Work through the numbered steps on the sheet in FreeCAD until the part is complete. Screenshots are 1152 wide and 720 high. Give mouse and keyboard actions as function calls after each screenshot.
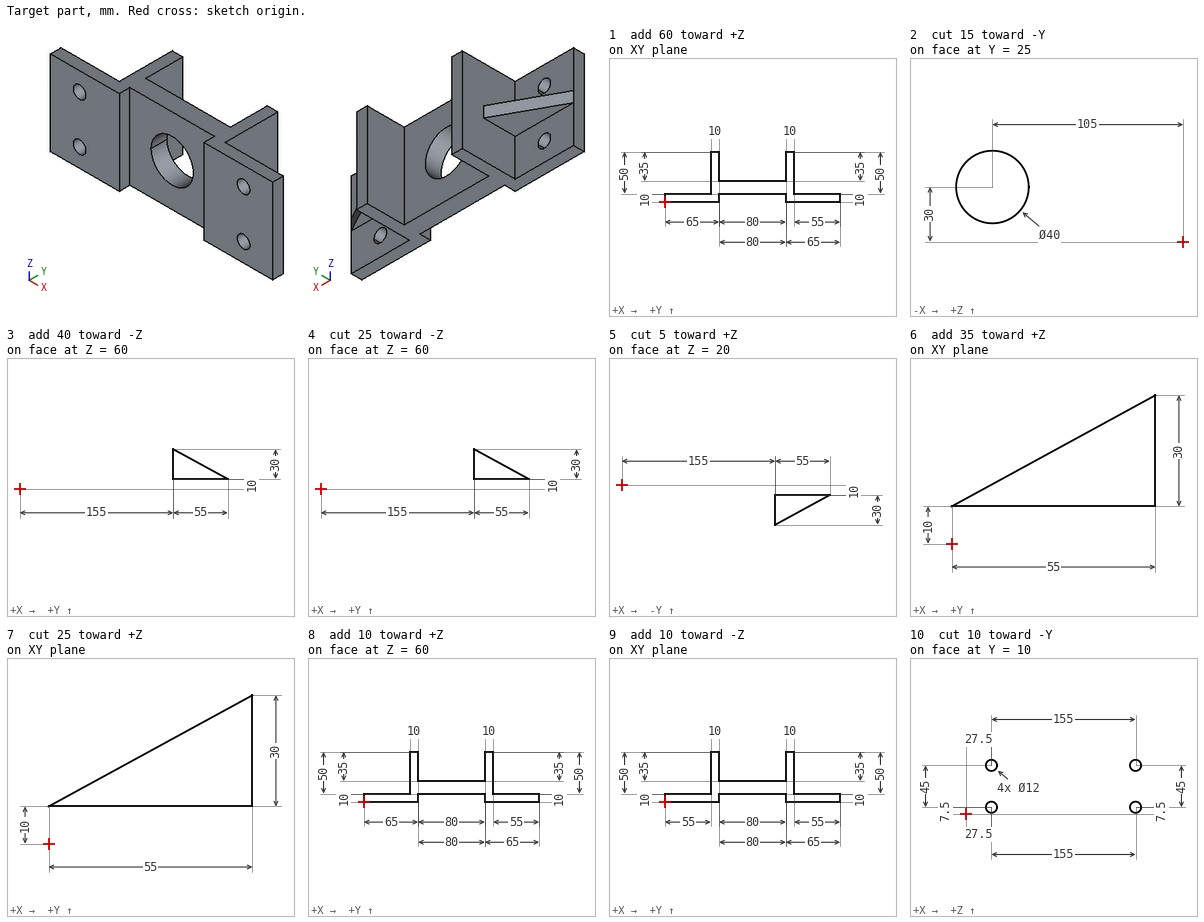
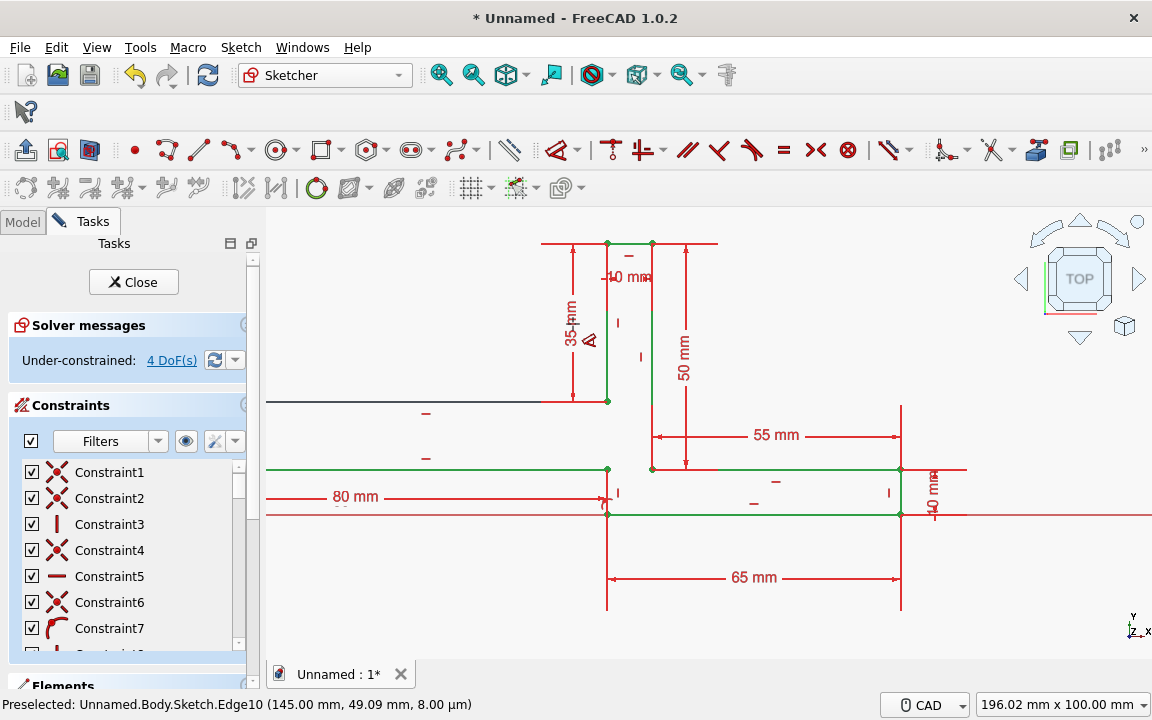
click(499, 402)
click(451, 436)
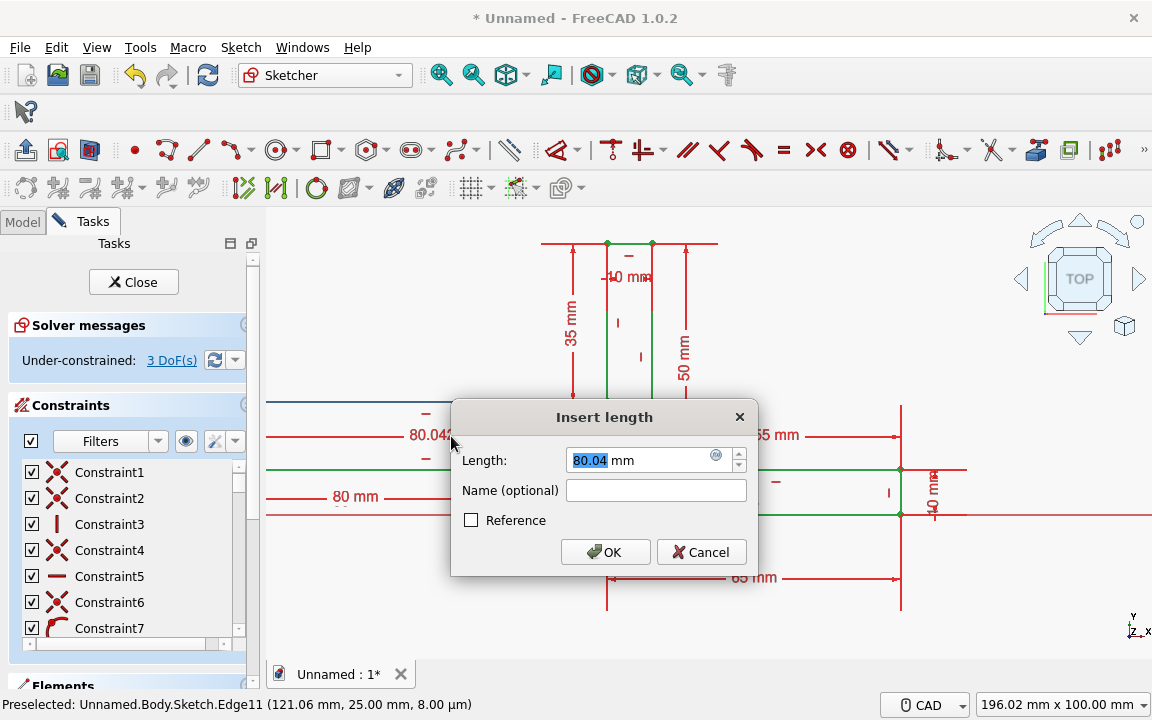
text(80)
key(Return)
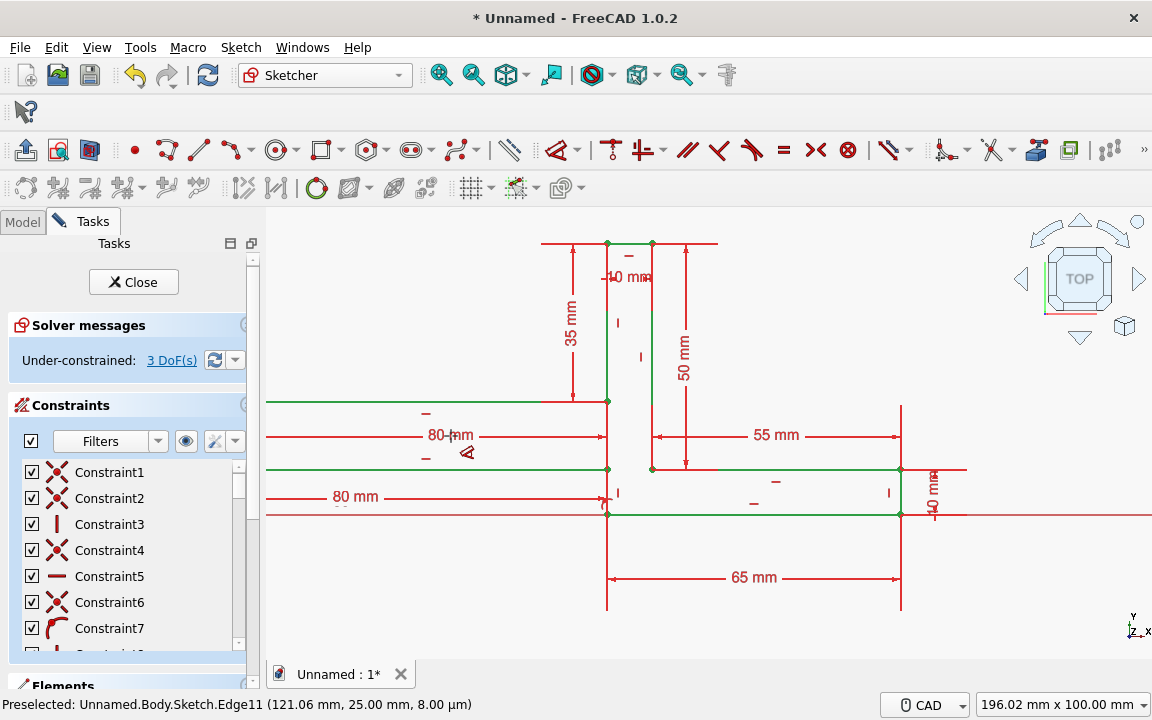
scroll(901, 498, down, 3)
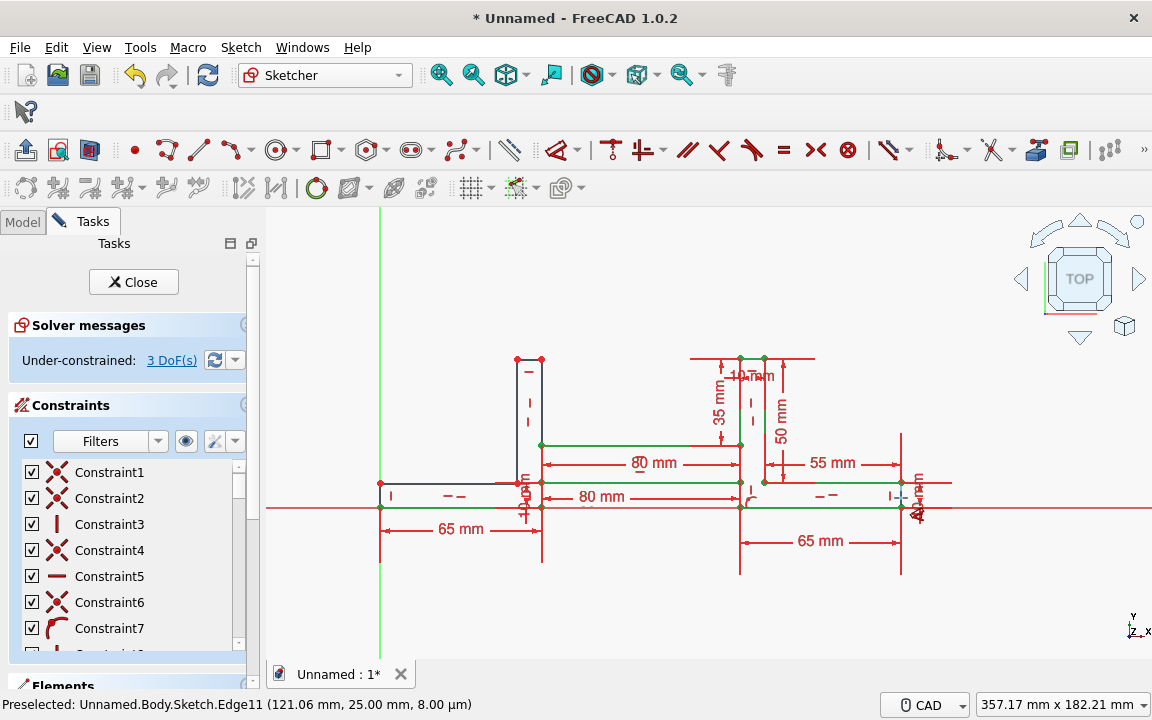
click(542, 420)
click(576, 403)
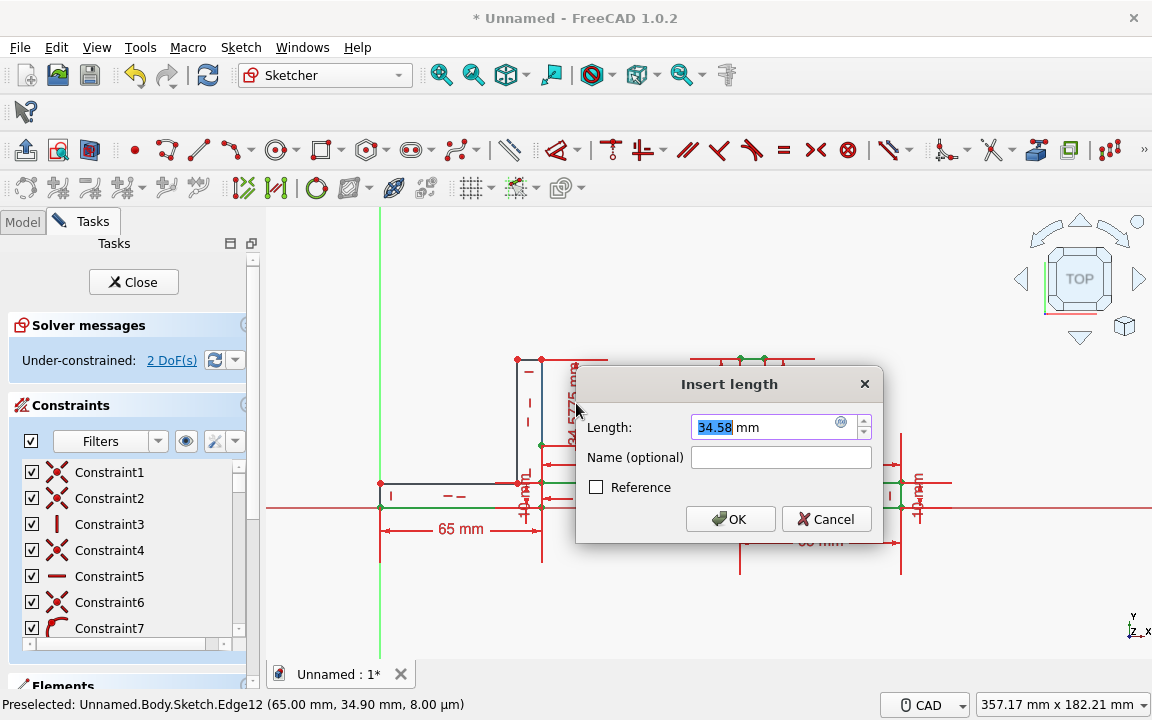
text(35)
key(Return)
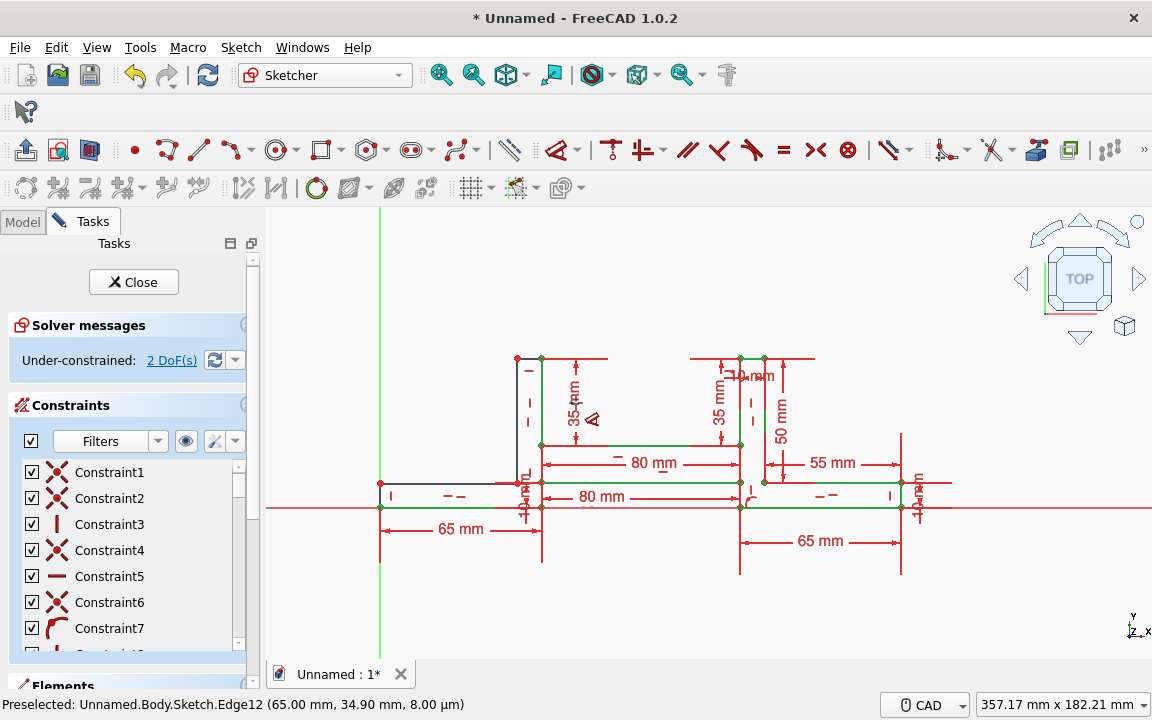
scroll(532, 359, up, 3)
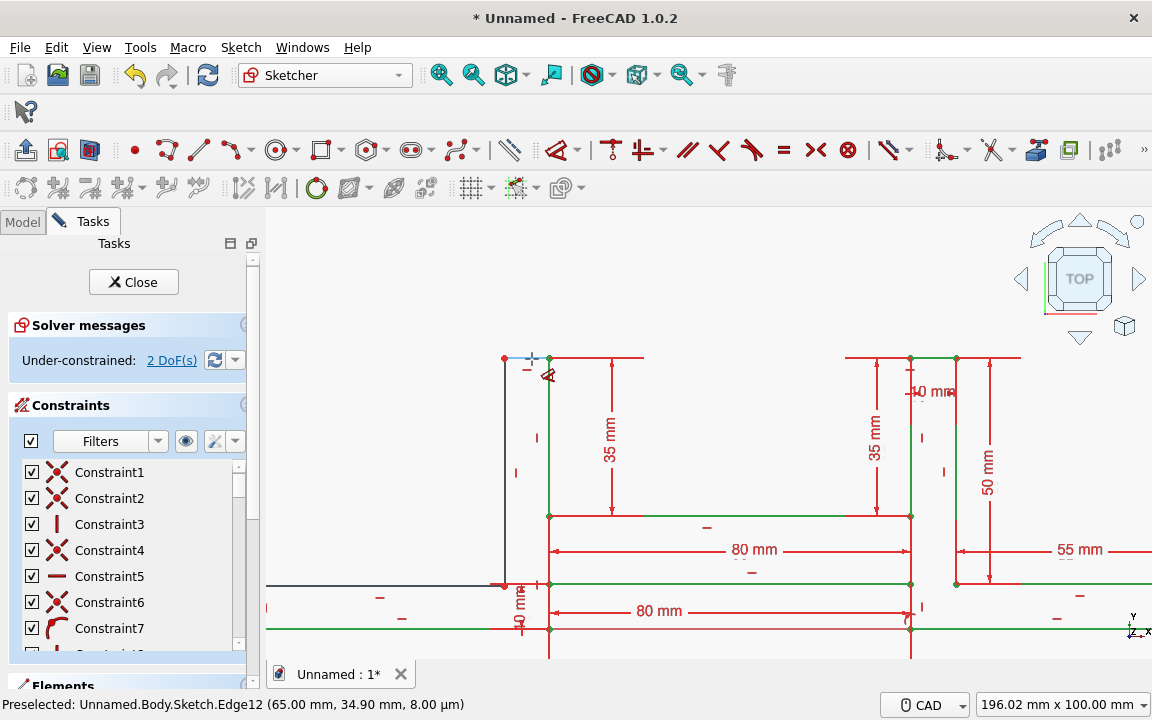
click(531, 358)
click(527, 324)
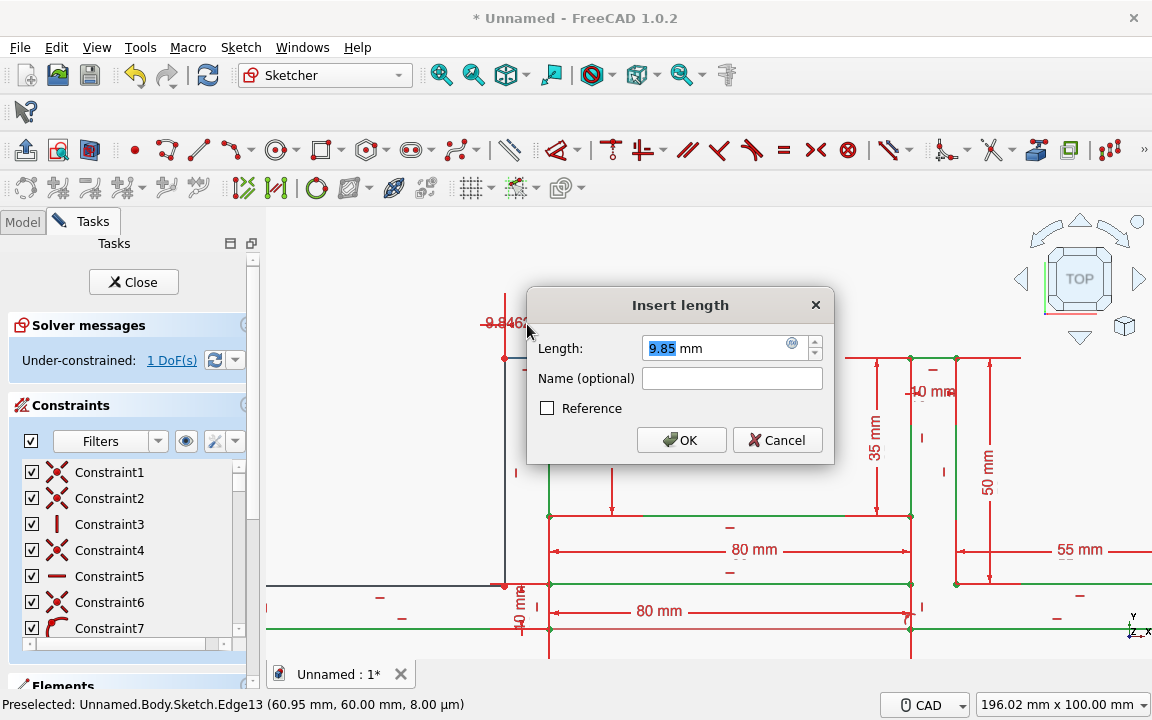
text(10)
key(Return)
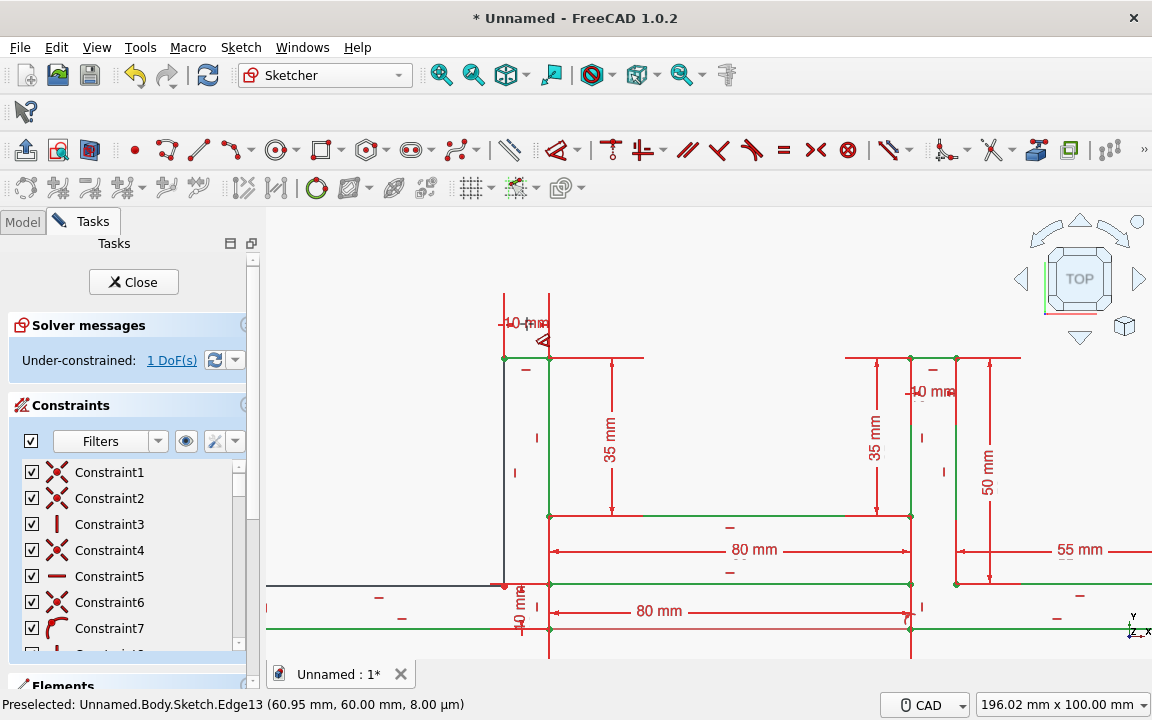
click(504, 427)
click(470, 472)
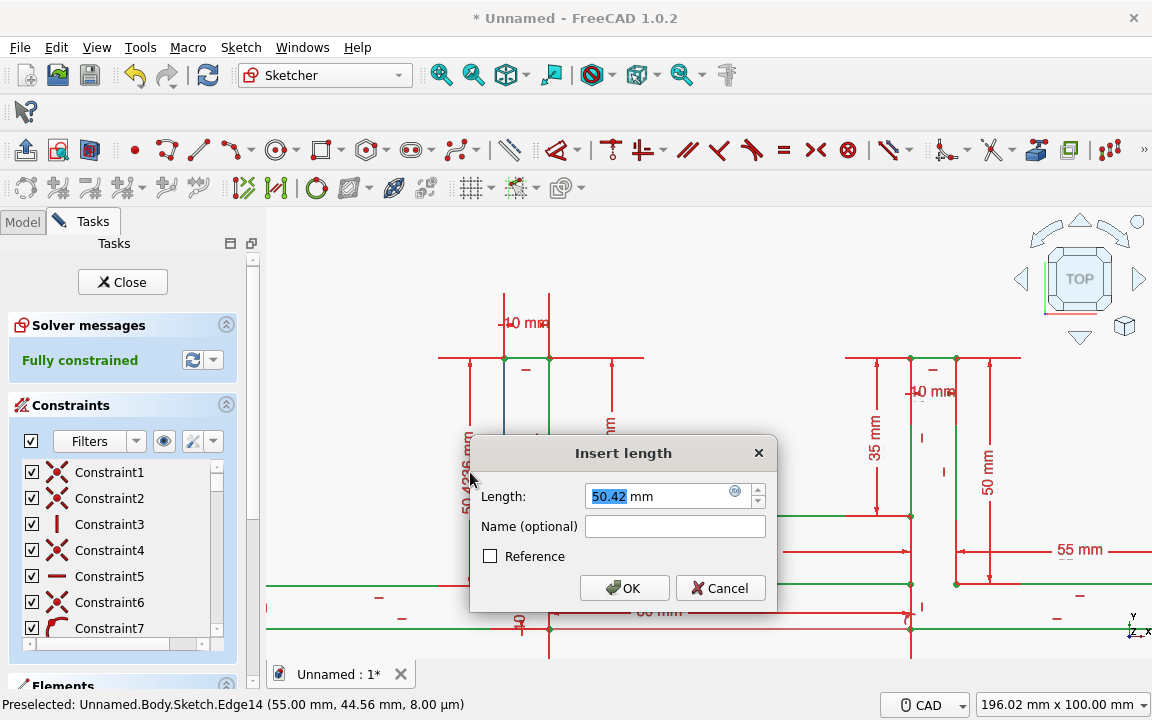
text(50)
key(Return)
key(Escape)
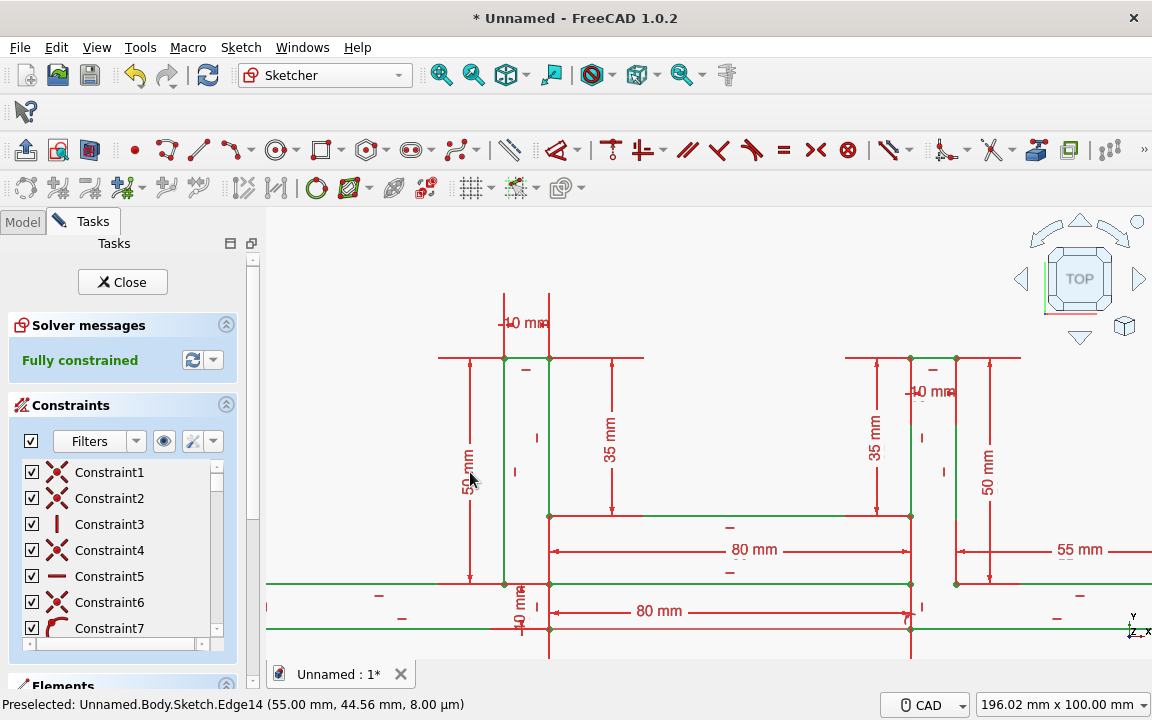
click(123, 282)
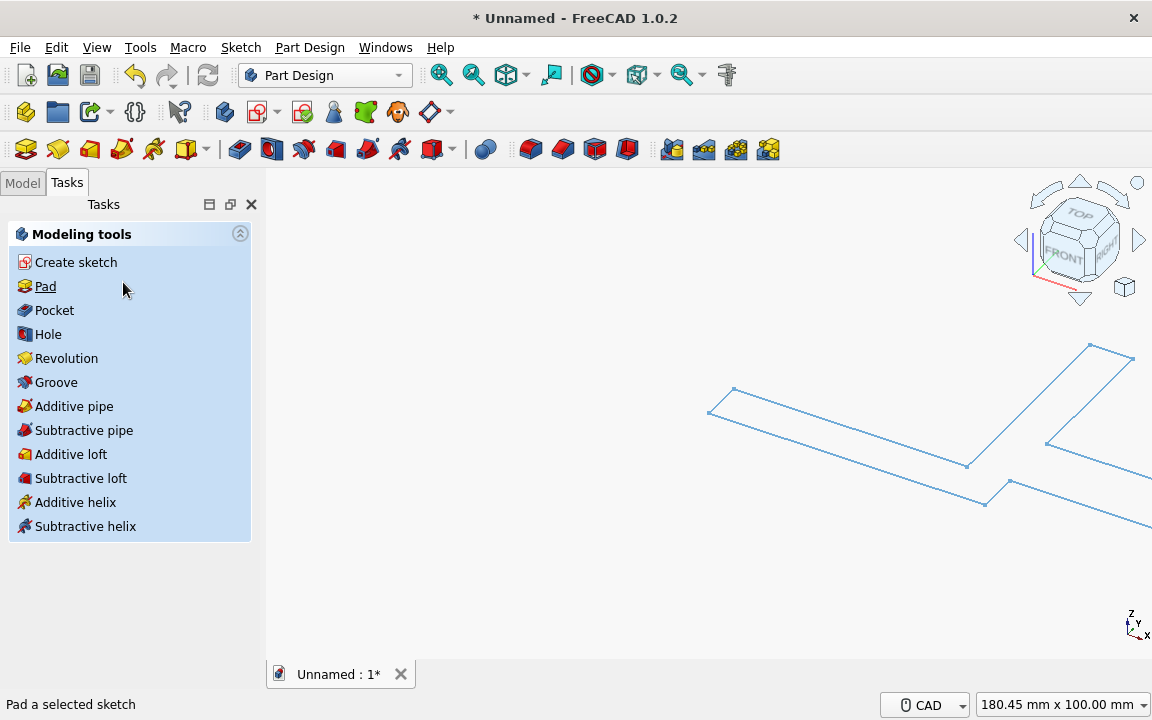
click(26, 150)